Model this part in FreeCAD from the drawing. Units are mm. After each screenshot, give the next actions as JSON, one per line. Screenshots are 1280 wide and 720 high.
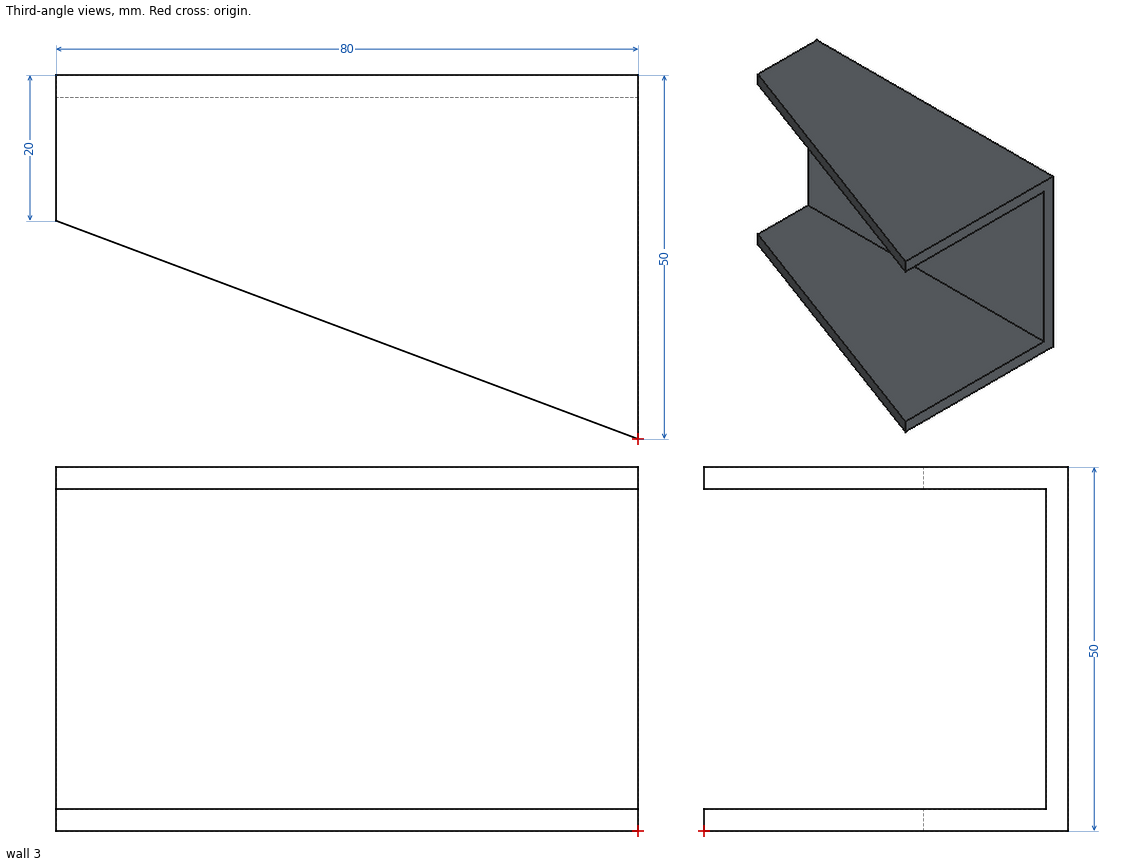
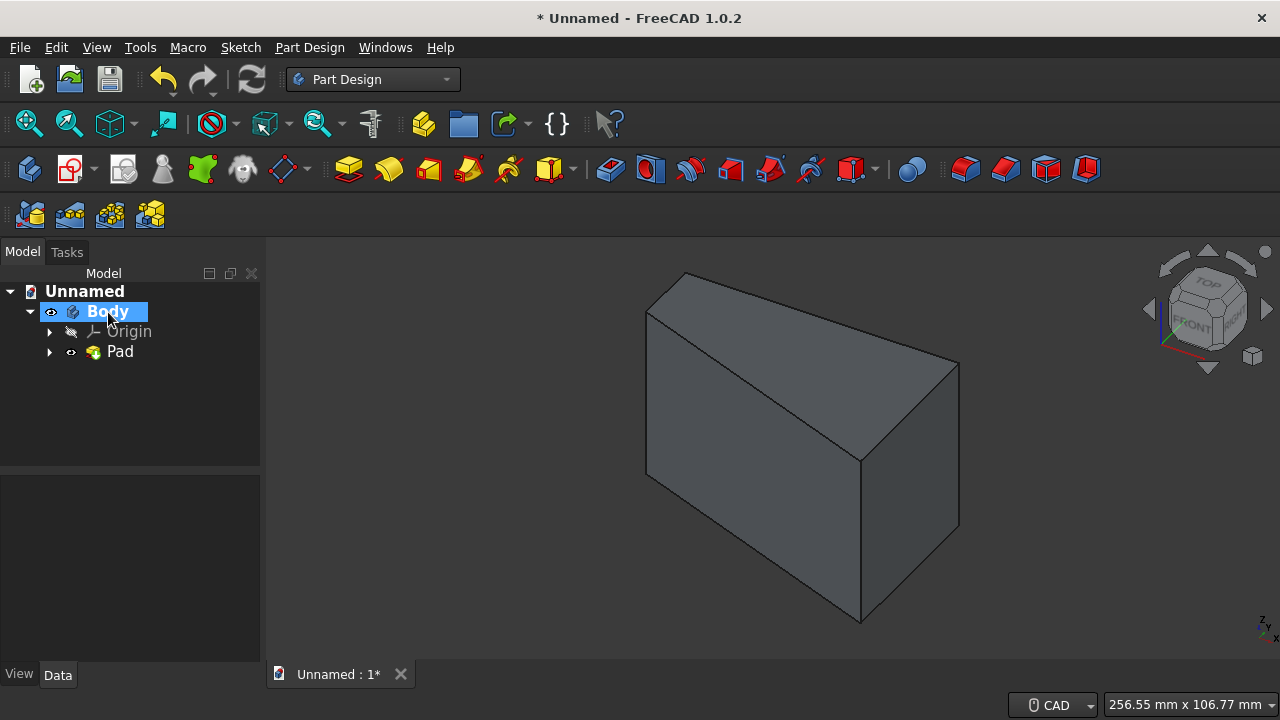
{"action": "left_click", "coordinate": [910, 492]}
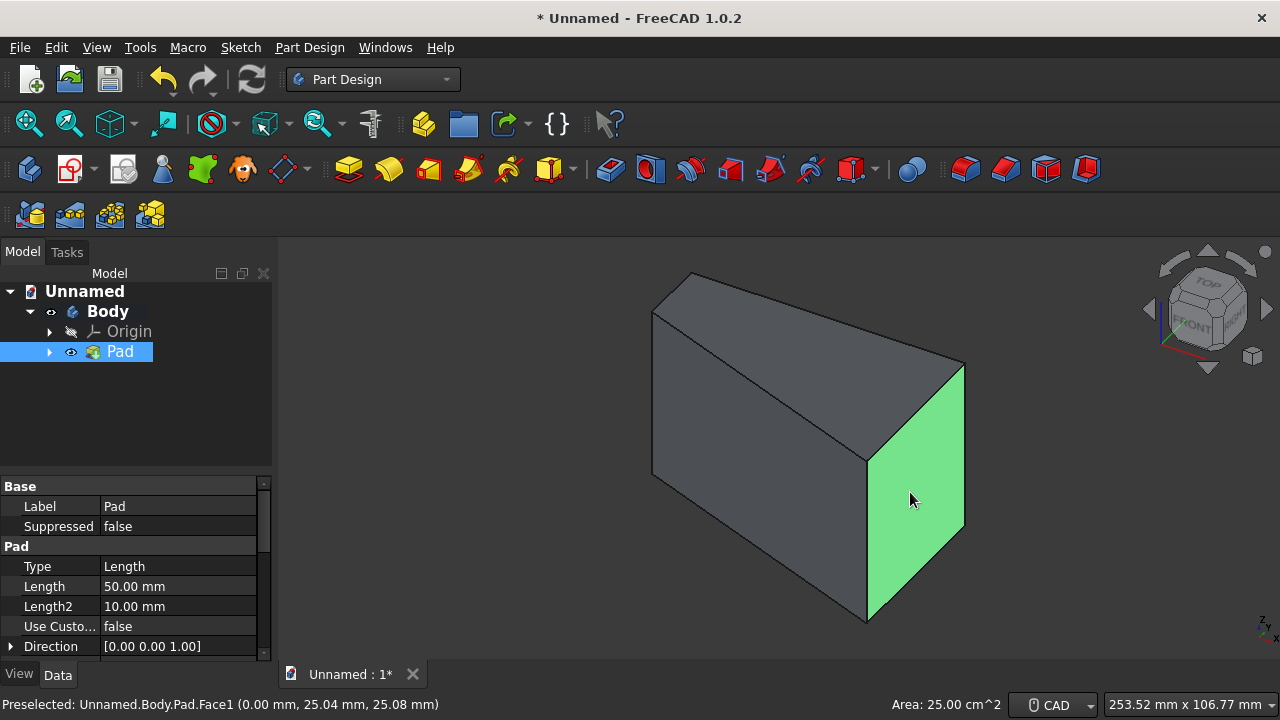
{"action": "left_click", "coordinate": [790, 488], "text": "ctrl"}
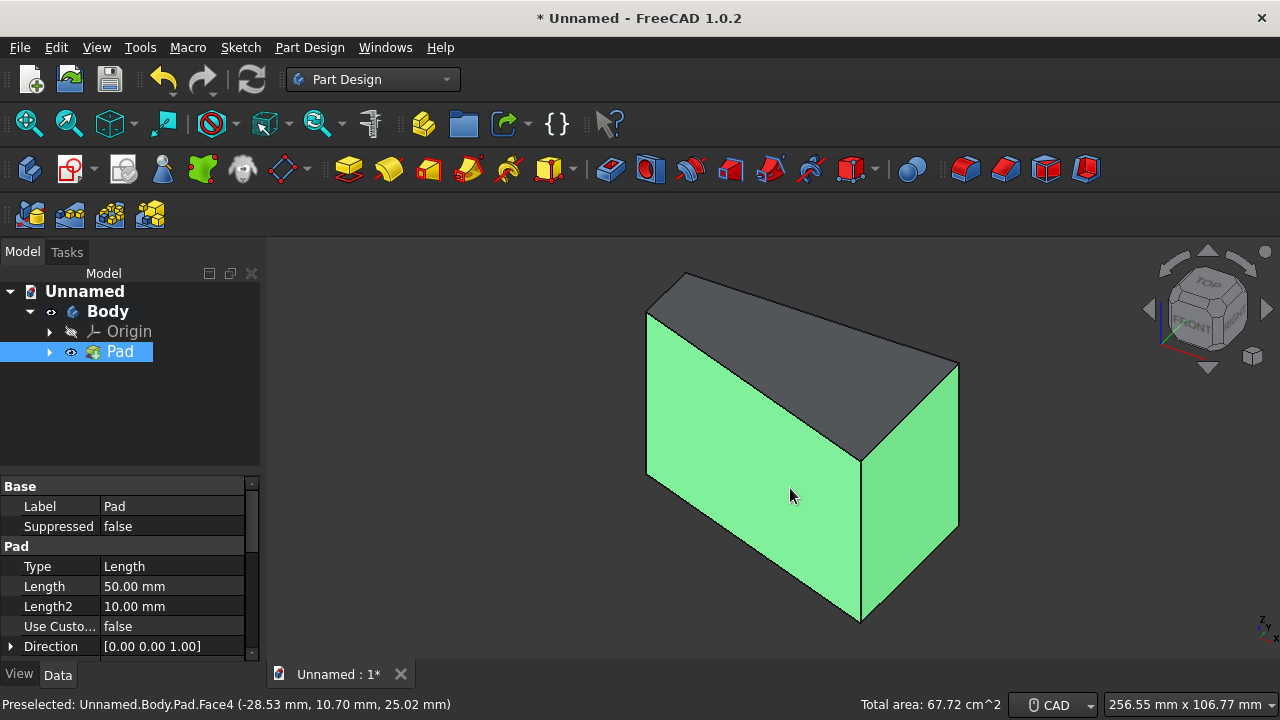
{"action": "key", "text": "0"}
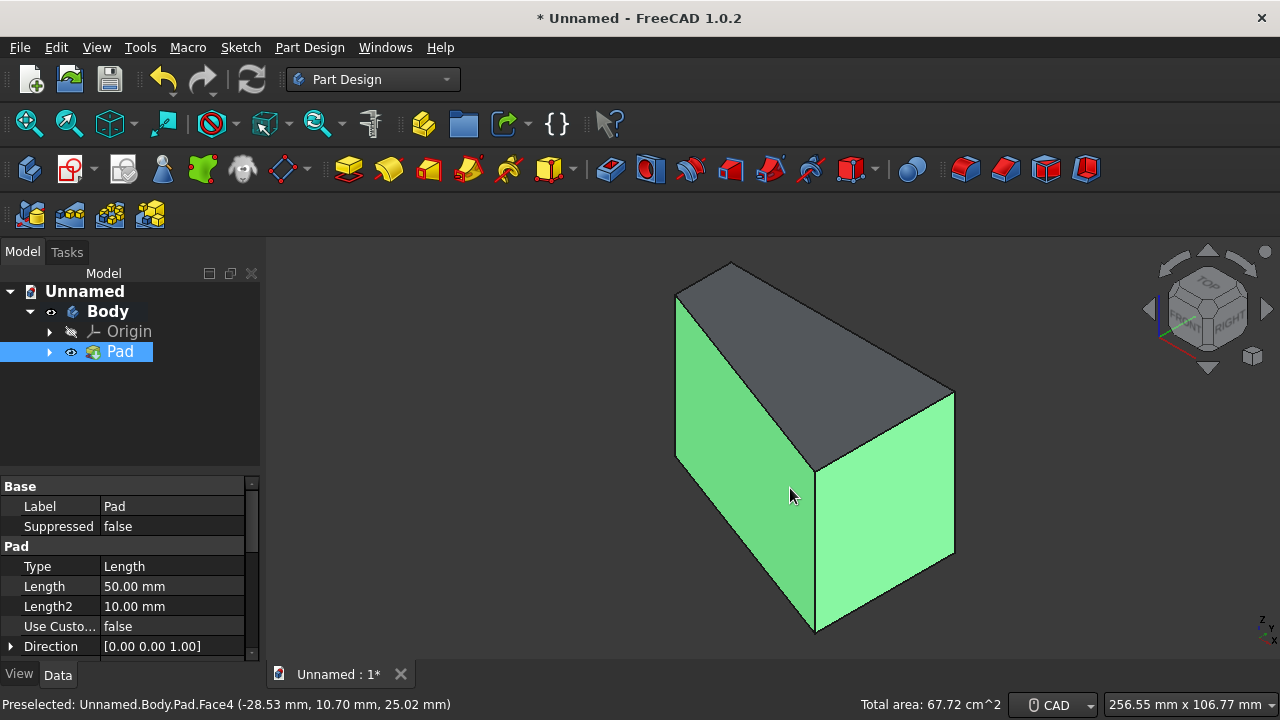
{"action": "key", "text": "2"}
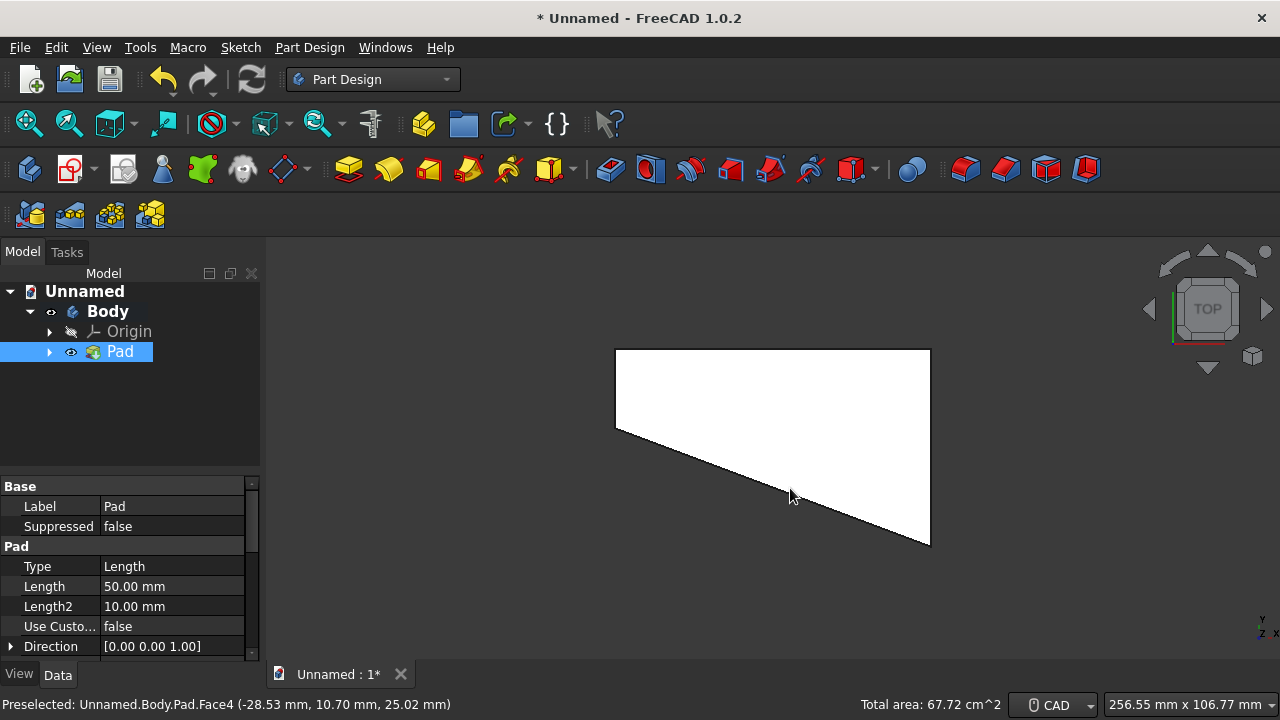
{"action": "key", "text": "1"}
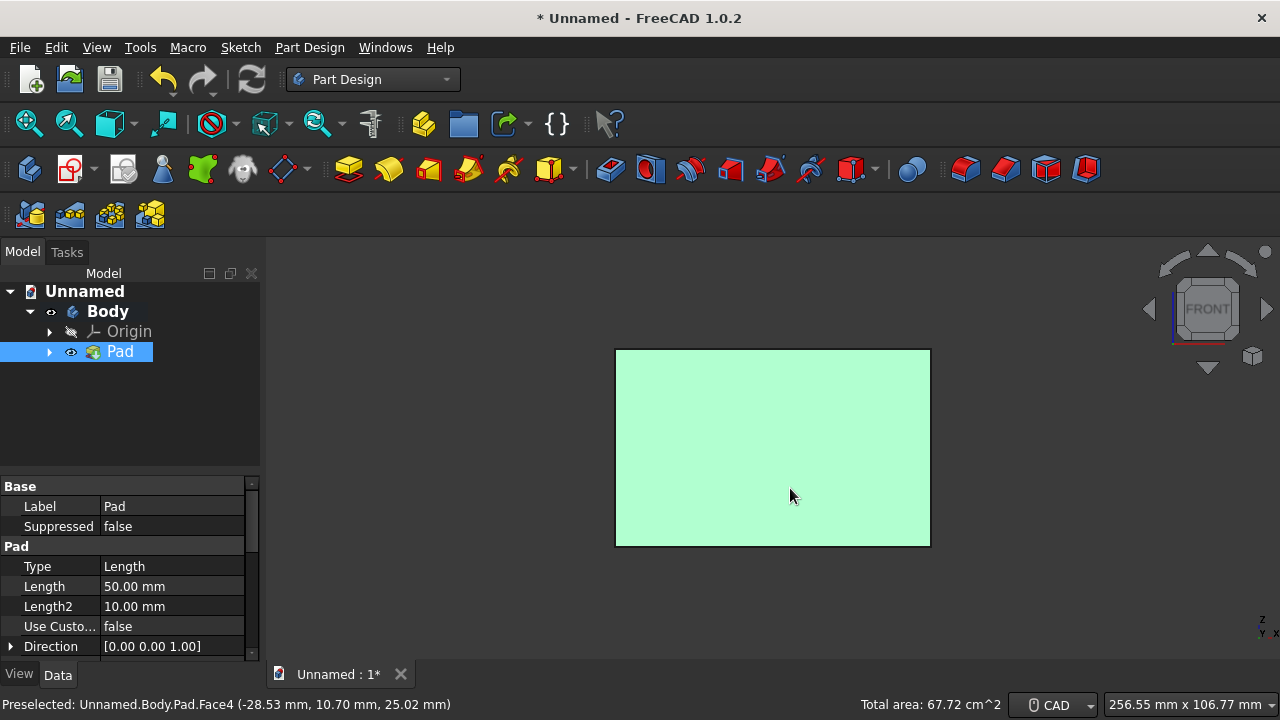
{"action": "key", "text": "3"}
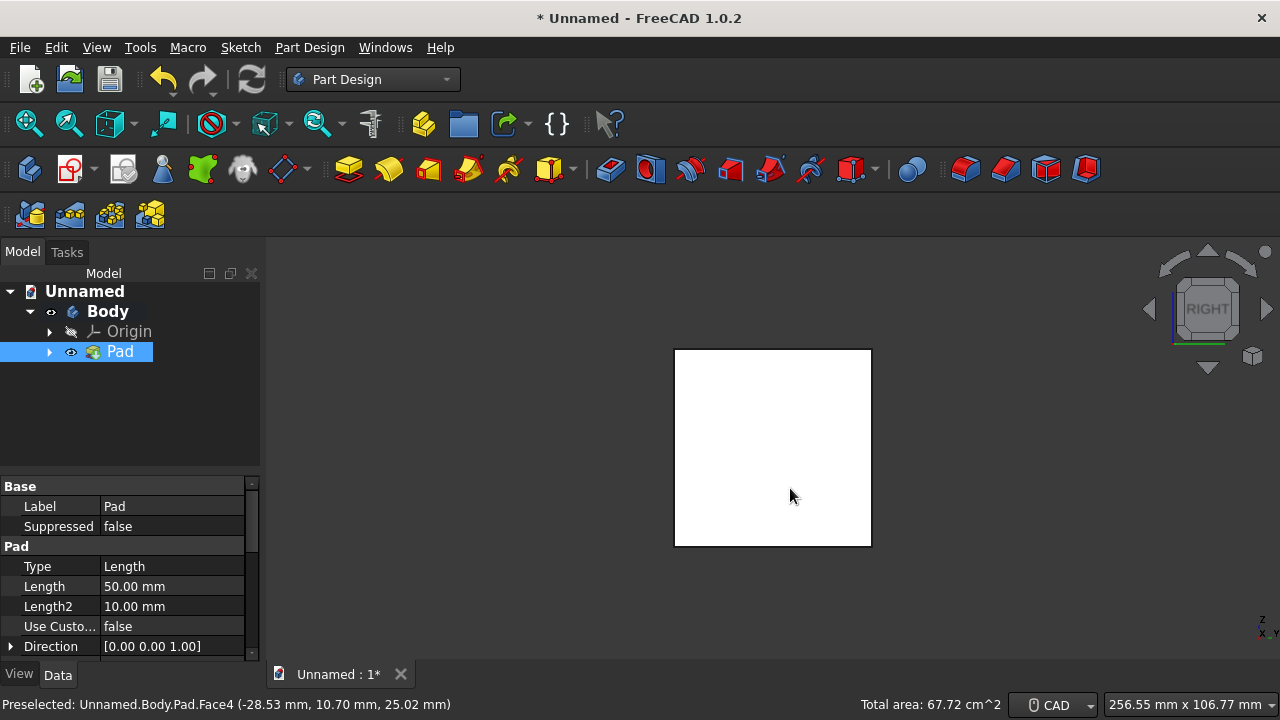
{"action": "key", "text": "5"}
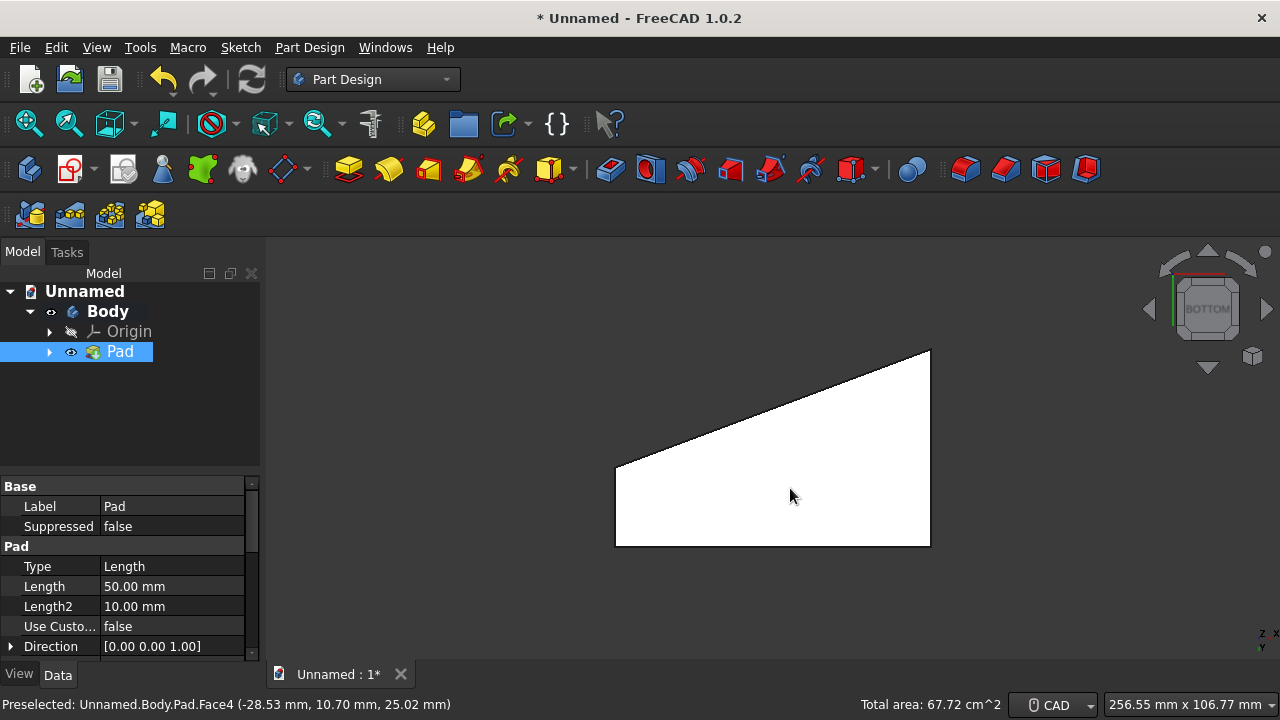
{"action": "key", "text": "4"}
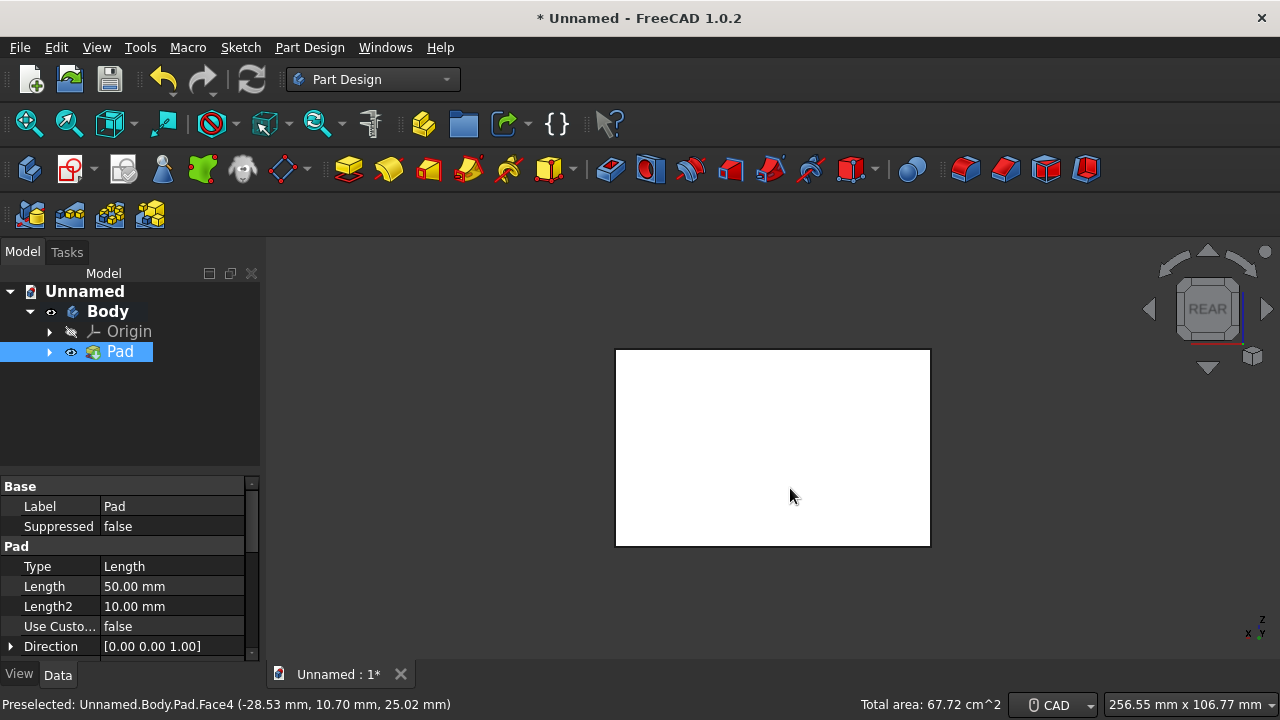
{"action": "key", "text": "6"}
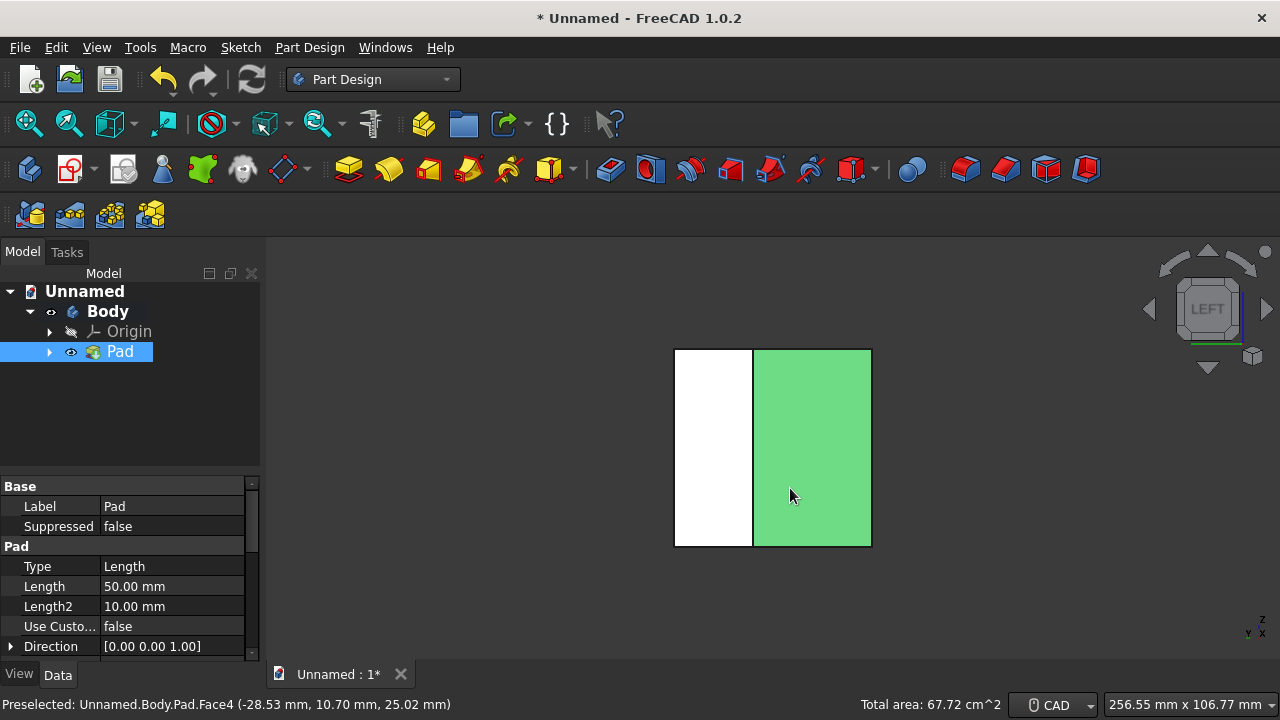
{"action": "left_click", "coordinate": [714, 391], "text": "ctrl"}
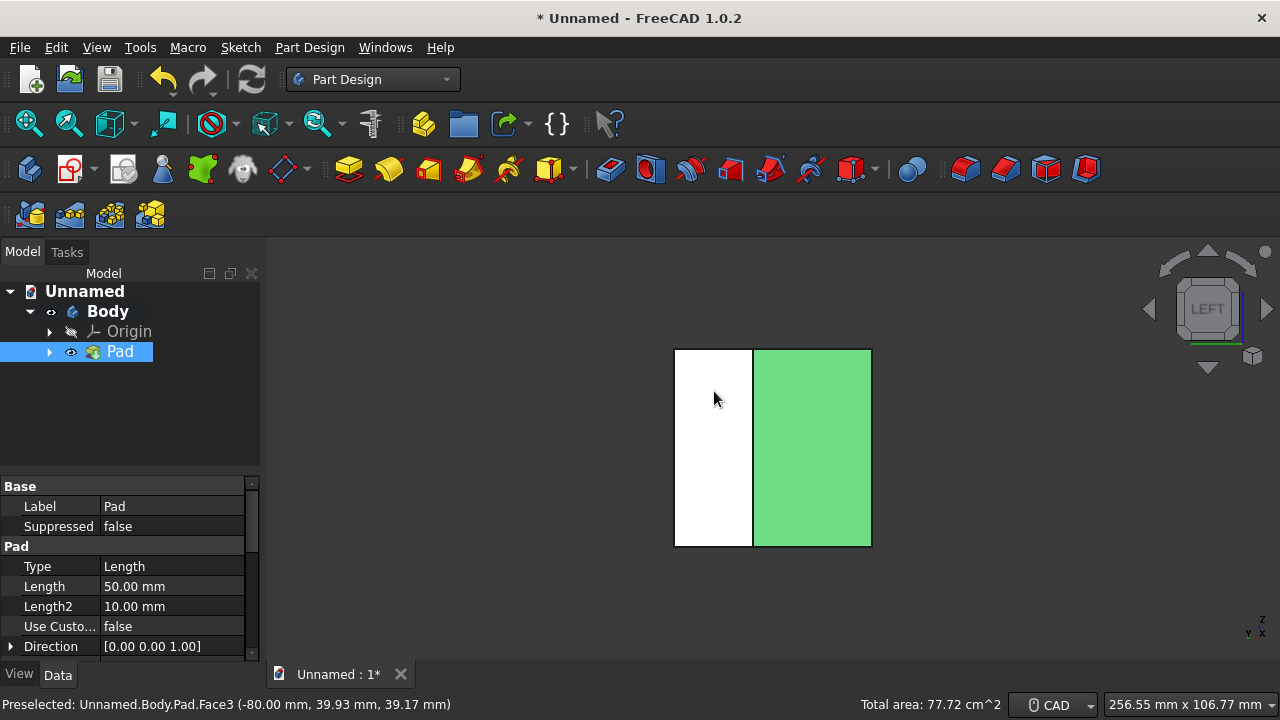
{"action": "left_click", "coordinate": [1086, 170]}